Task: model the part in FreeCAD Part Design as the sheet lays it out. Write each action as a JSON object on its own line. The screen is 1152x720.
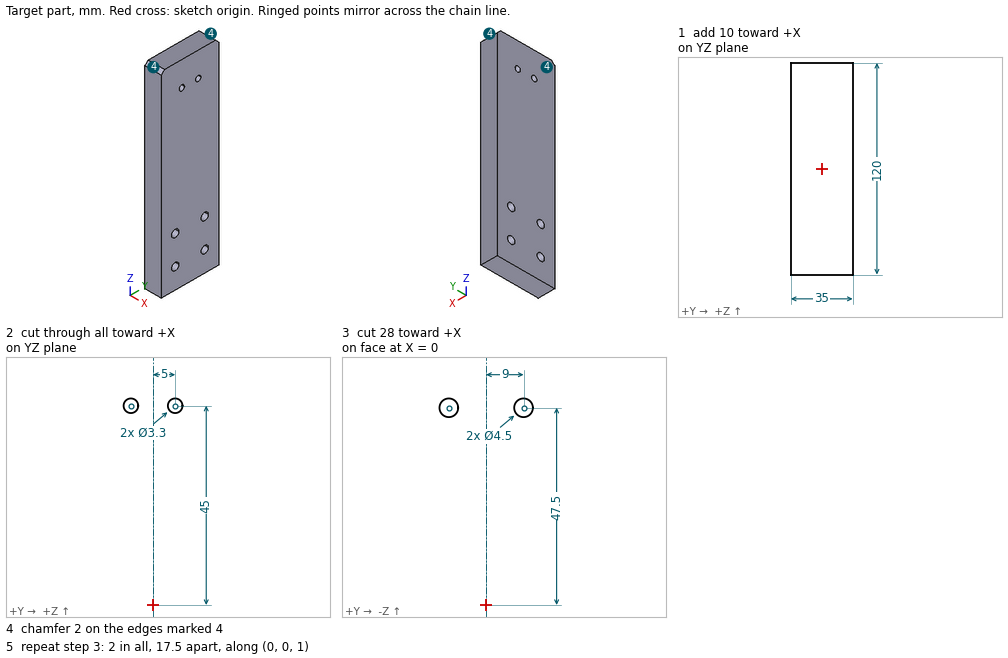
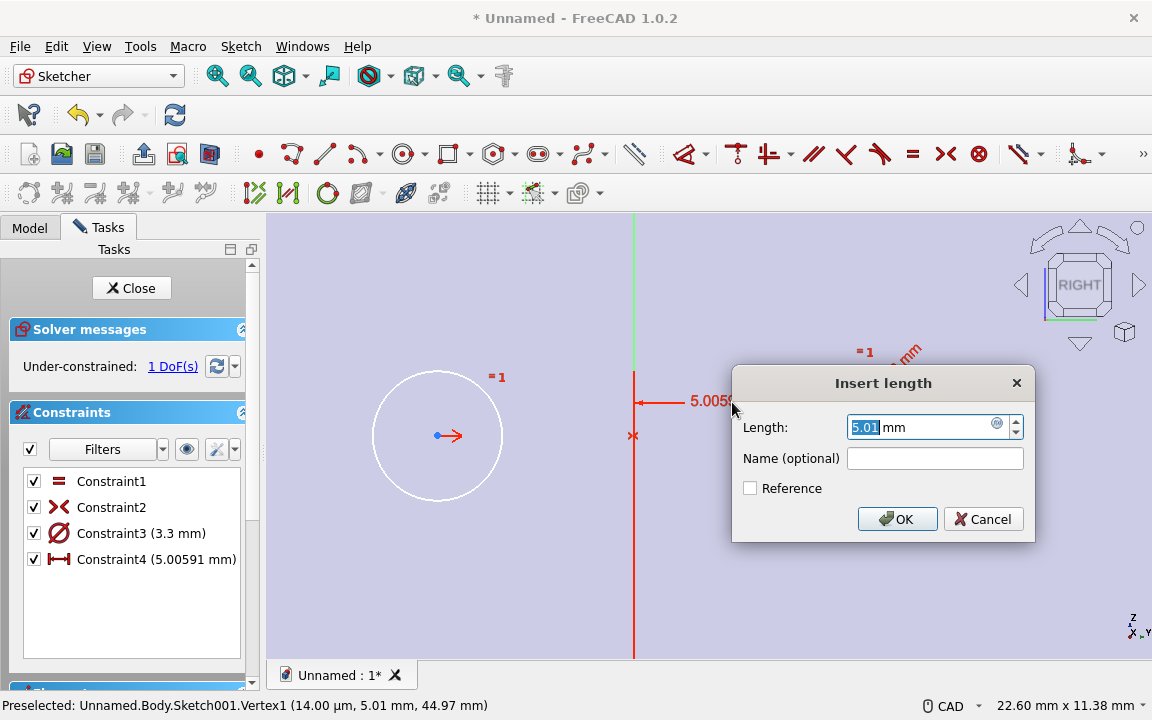
{"action": "type", "text": "5"}
{"action": "key", "text": "Return"}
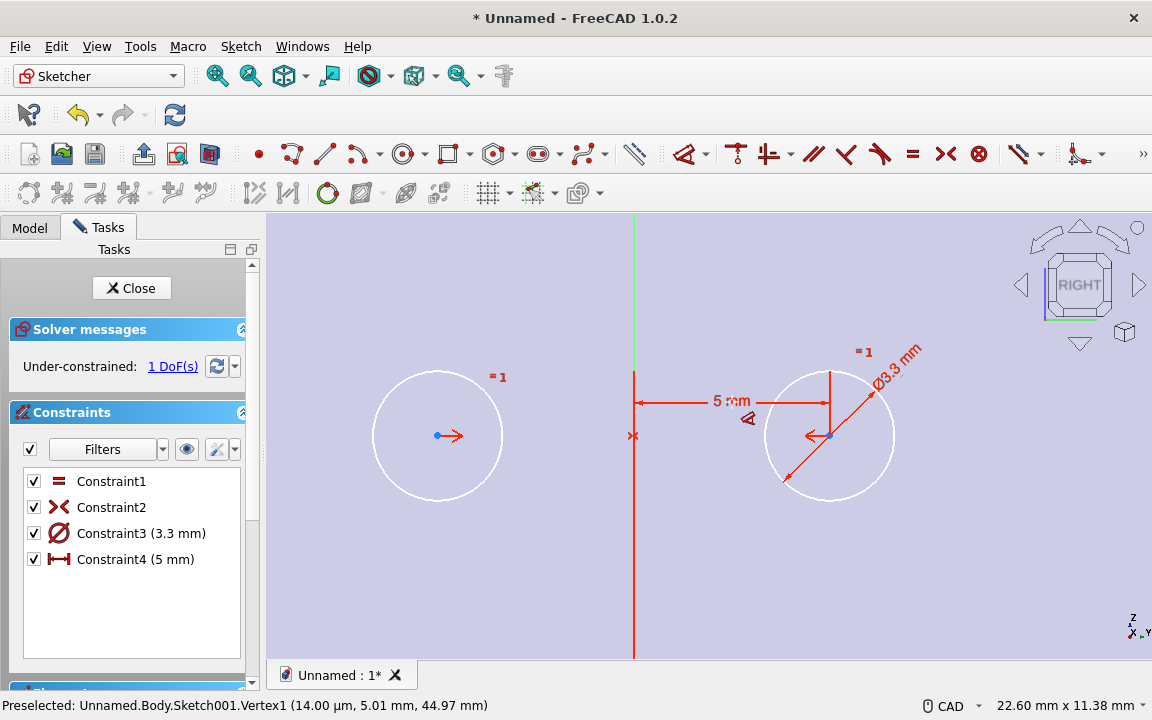
{"action": "left_click", "coordinate": [830, 436]}
{"action": "left_click", "coordinate": [864, 533]}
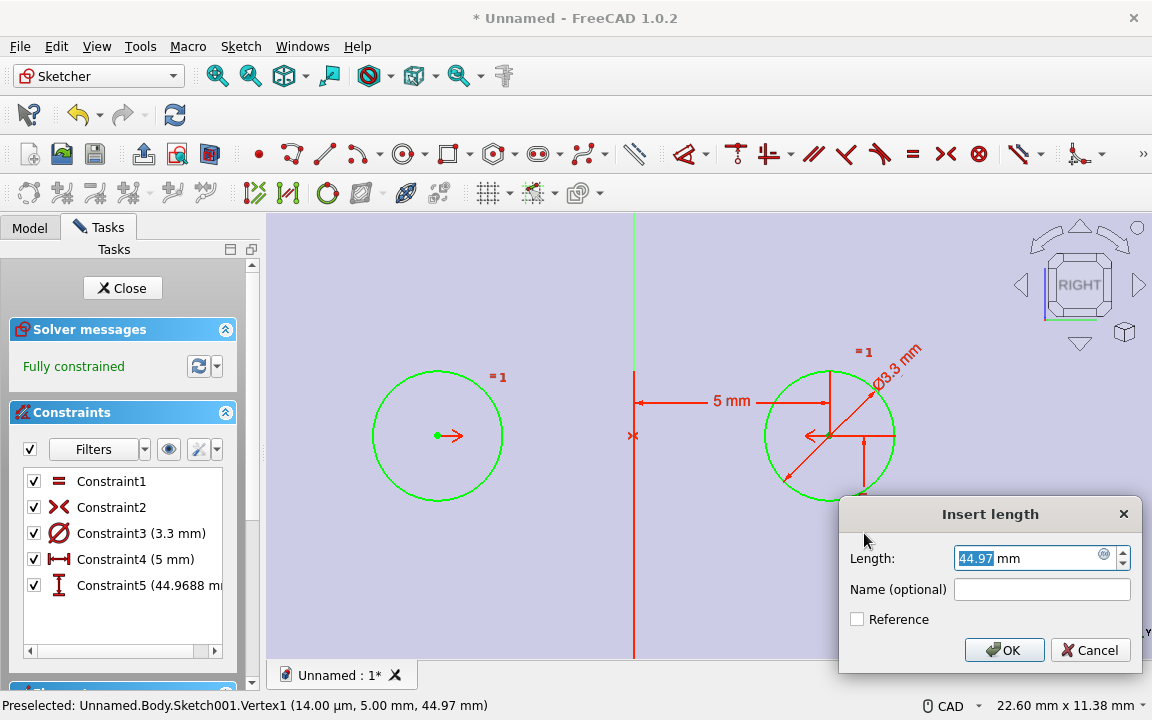
{"action": "type", "text": "45"}
{"action": "key", "text": "Return"}
{"action": "key", "text": "Escape"}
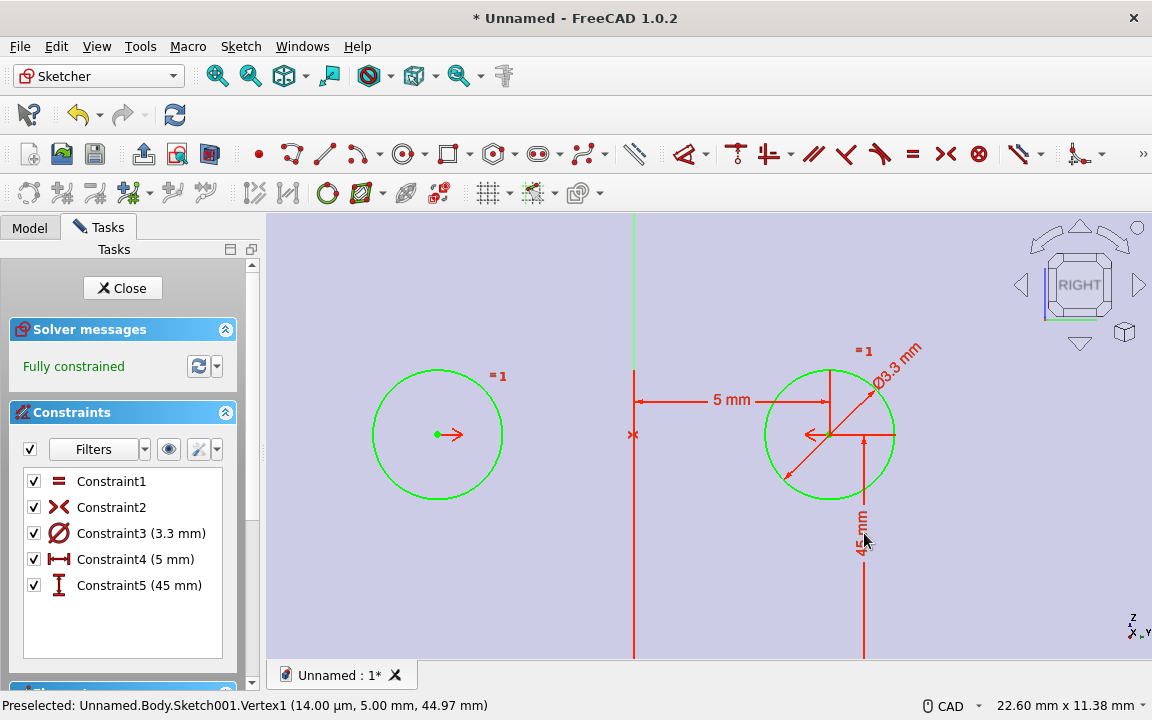
{"action": "left_click", "coordinate": [123, 288]}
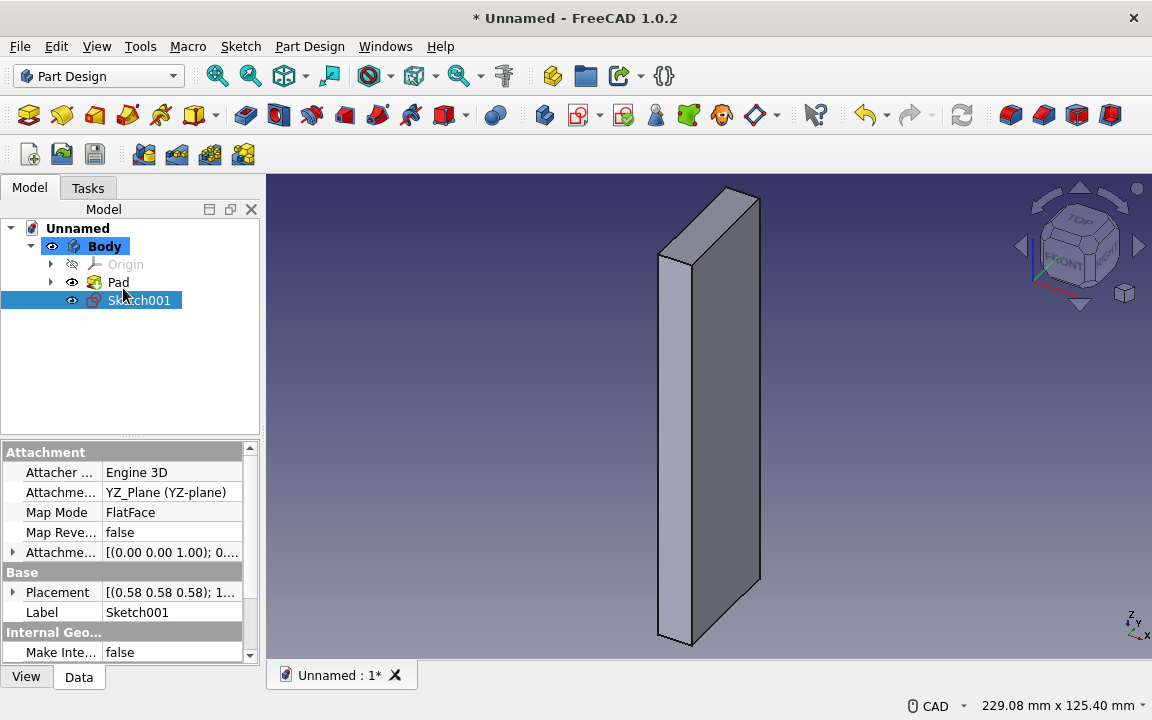
{"action": "left_click", "coordinate": [246, 116]}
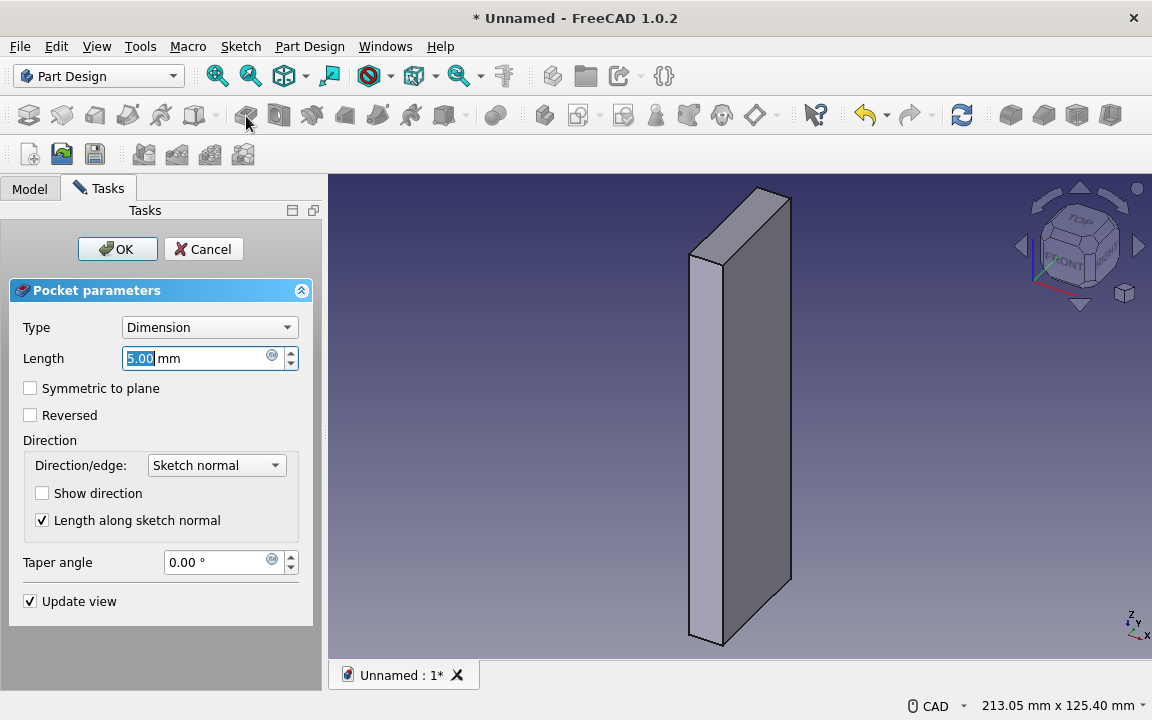
{"action": "left_click", "coordinate": [210, 328]}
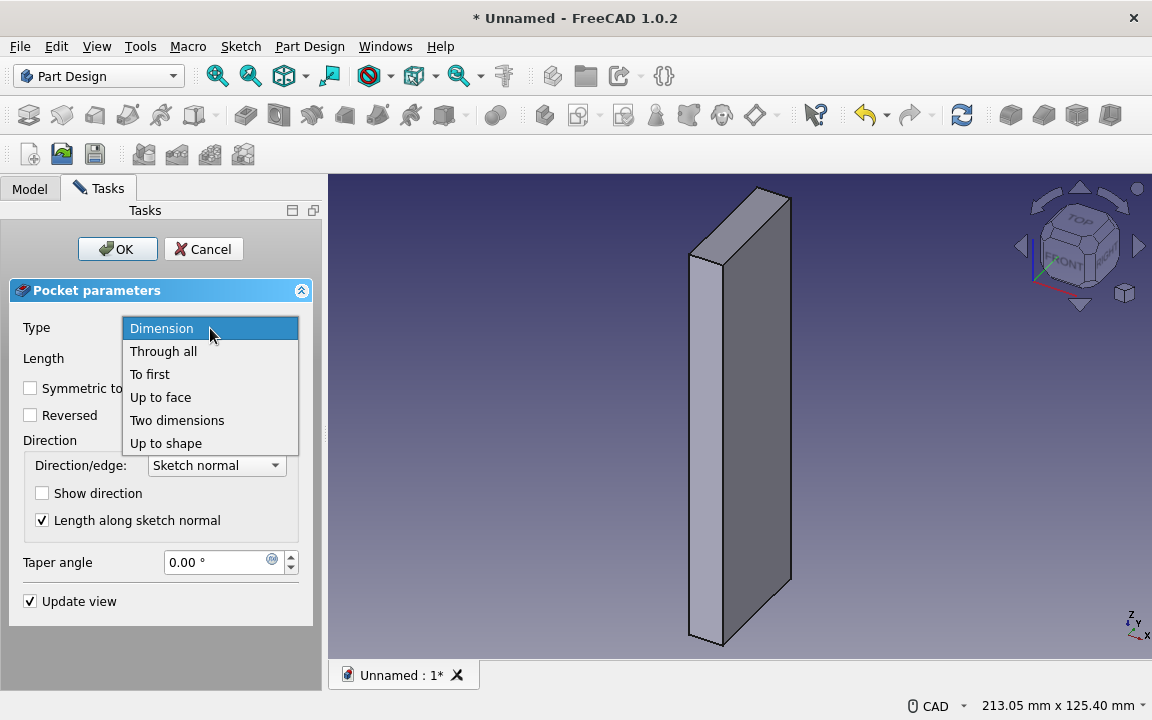
{"action": "left_click", "coordinate": [208, 352]}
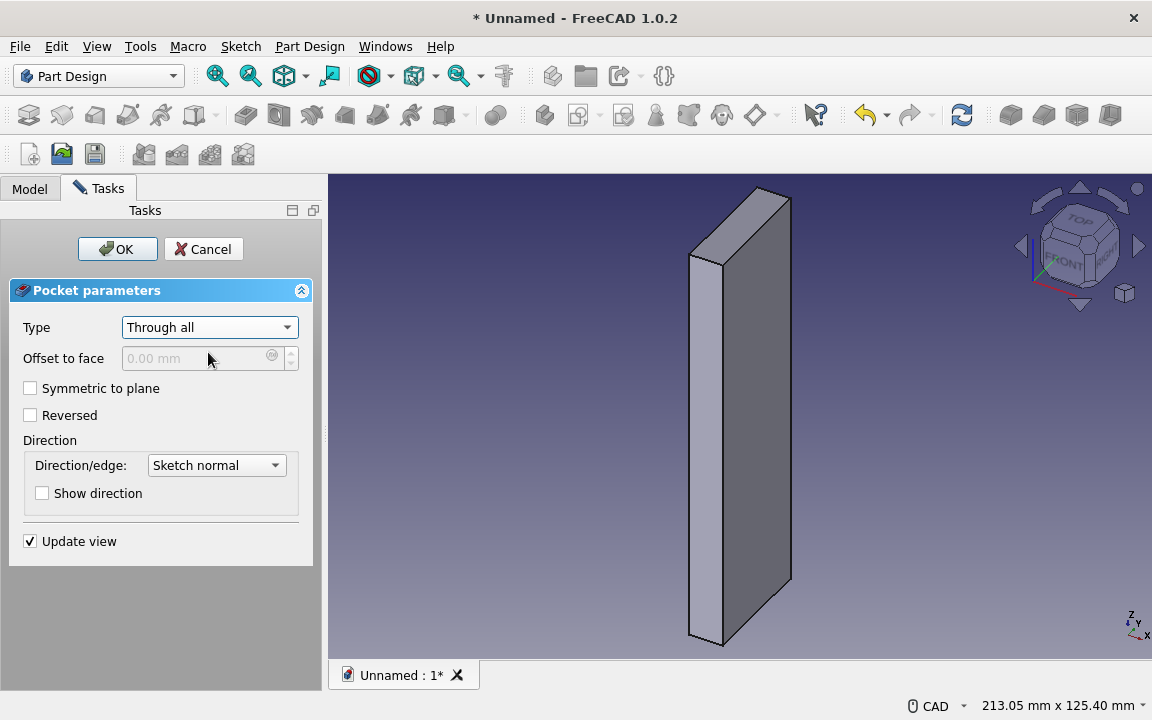
{"action": "left_click", "coordinate": [31, 415]}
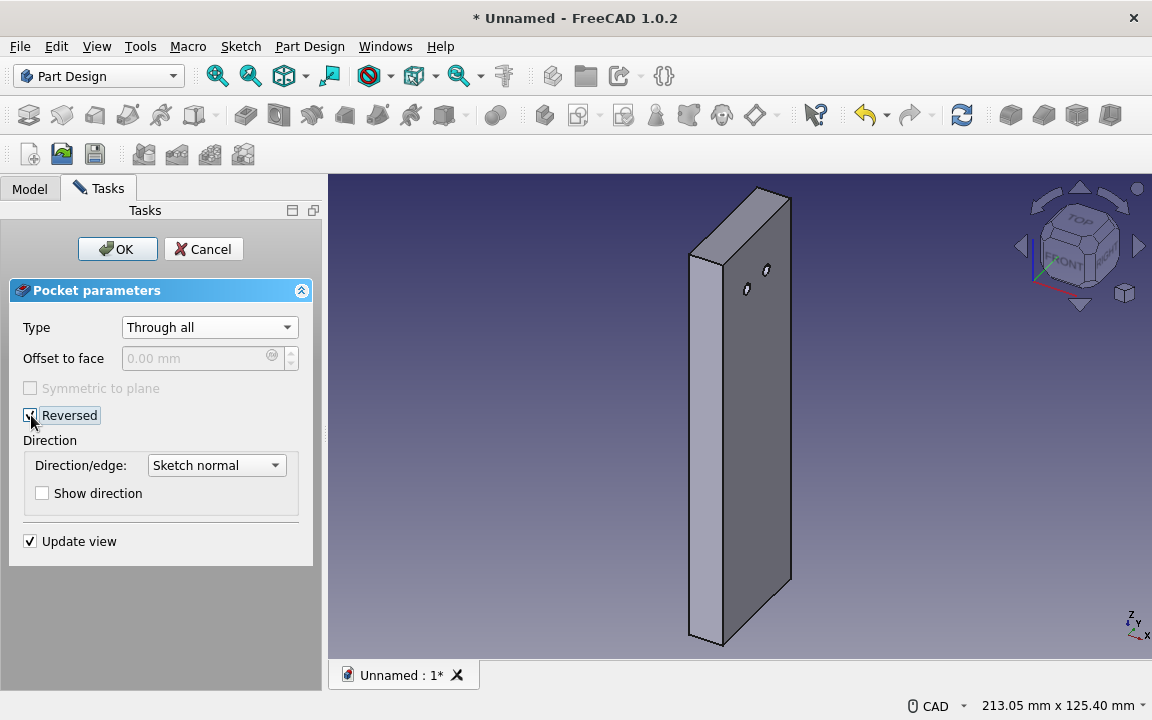
{"action": "left_click", "coordinate": [118, 249]}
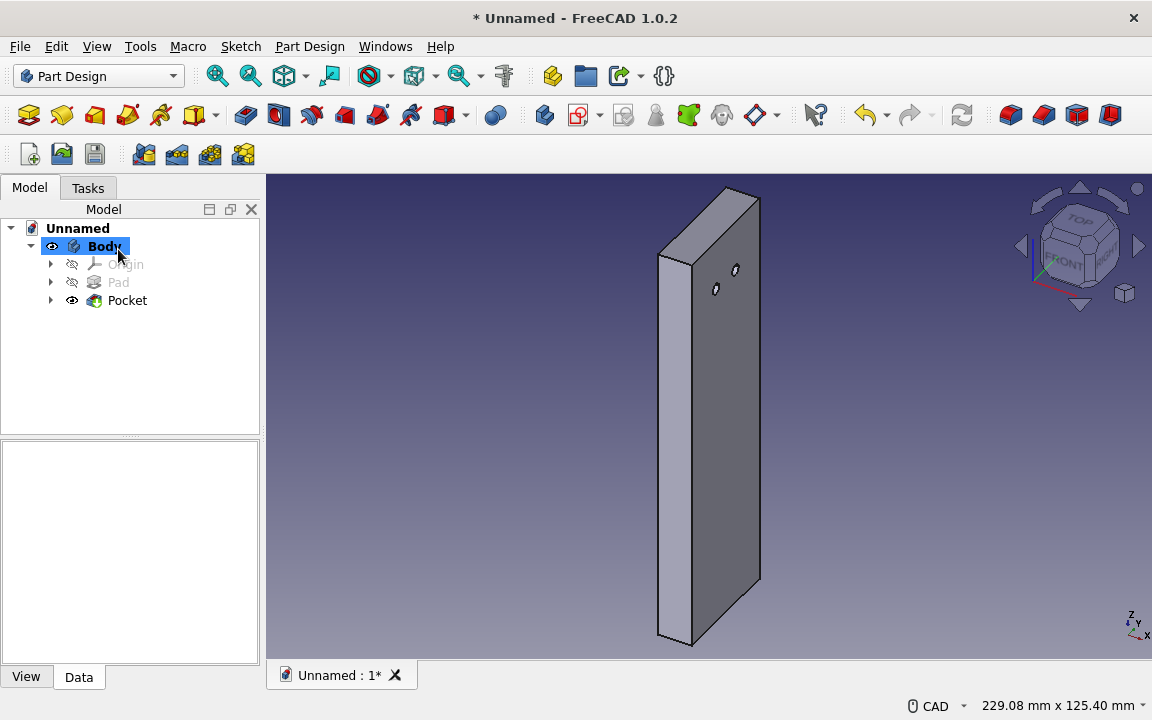
{"action": "key", "text": "6"}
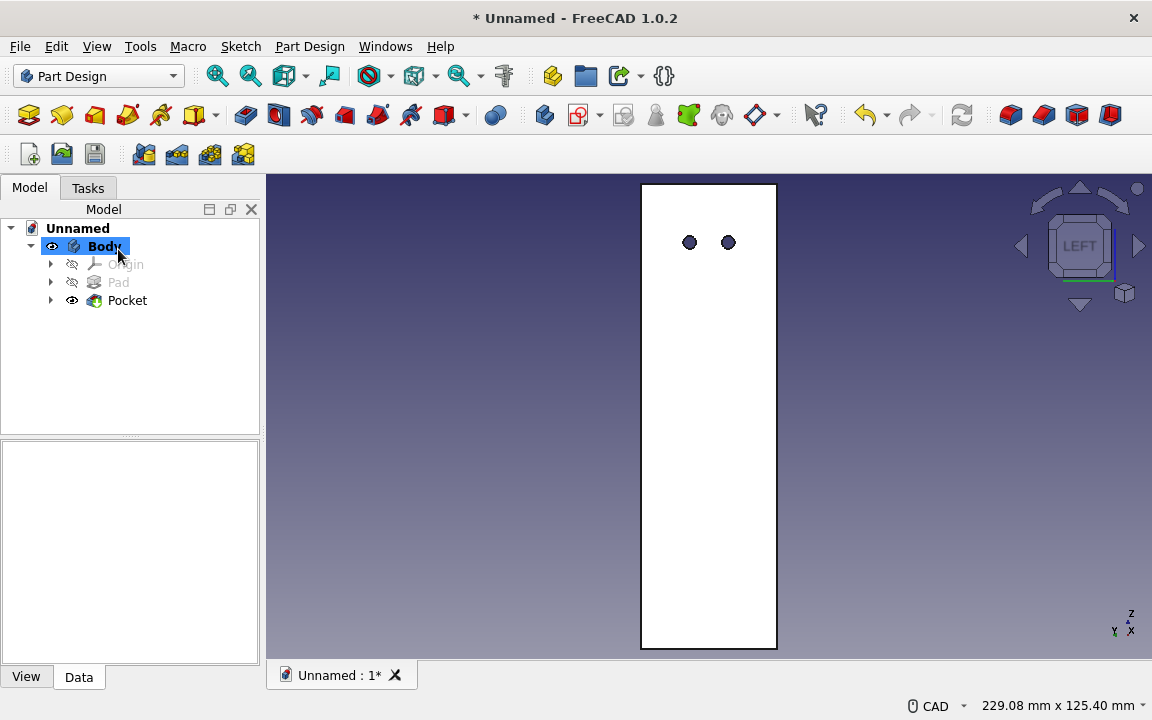
{"action": "left_click", "coordinate": [709, 548]}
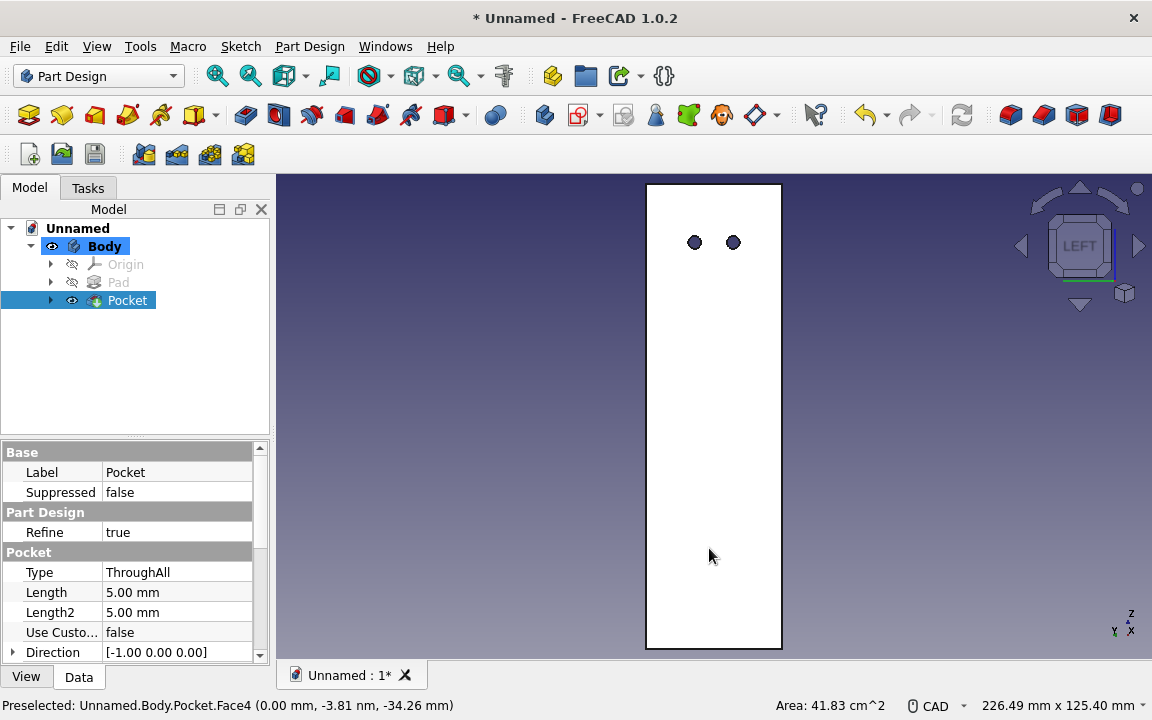
{"action": "left_click", "coordinate": [578, 116]}